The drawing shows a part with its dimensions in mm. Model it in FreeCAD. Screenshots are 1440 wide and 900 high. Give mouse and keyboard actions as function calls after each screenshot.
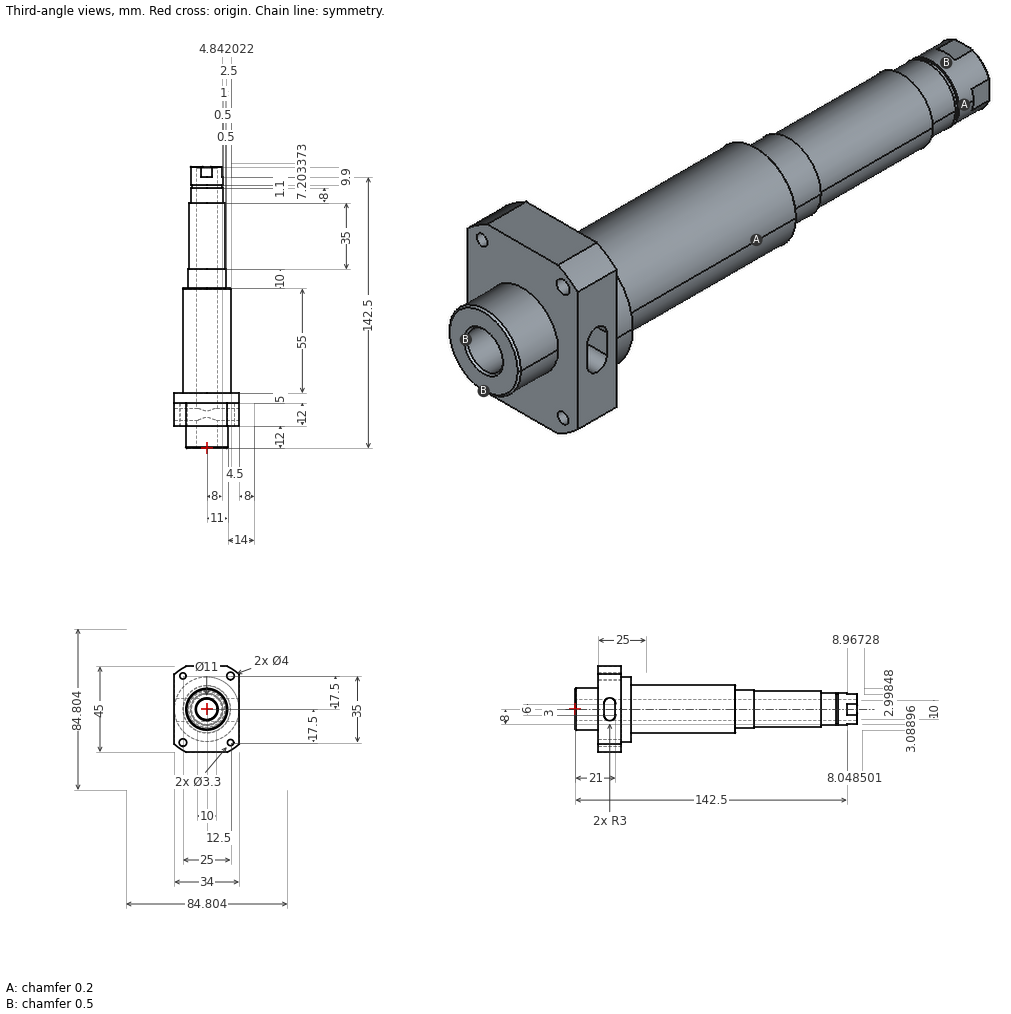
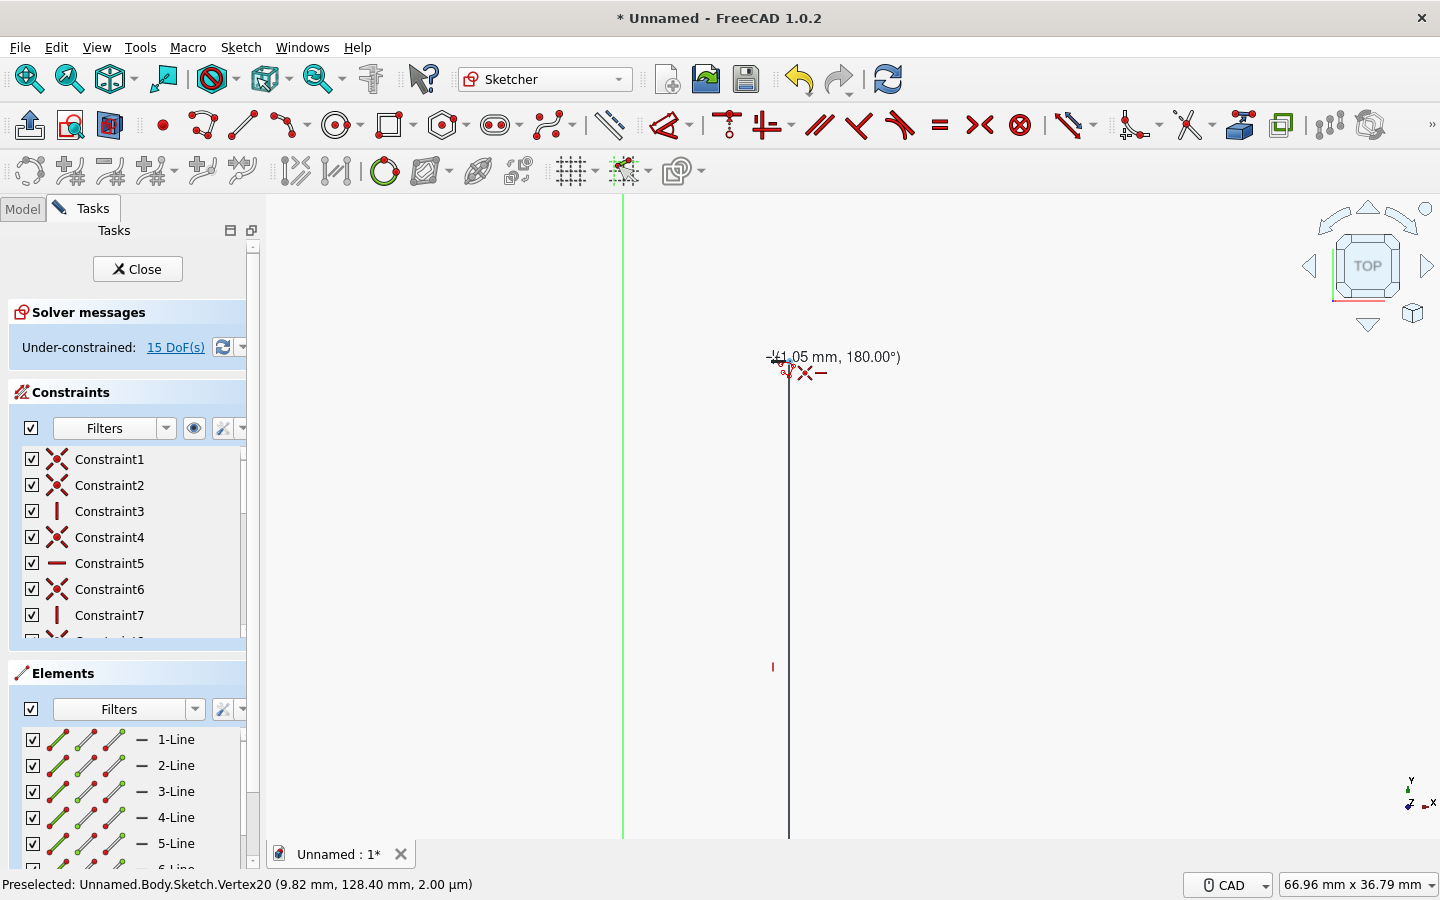
click(772, 356)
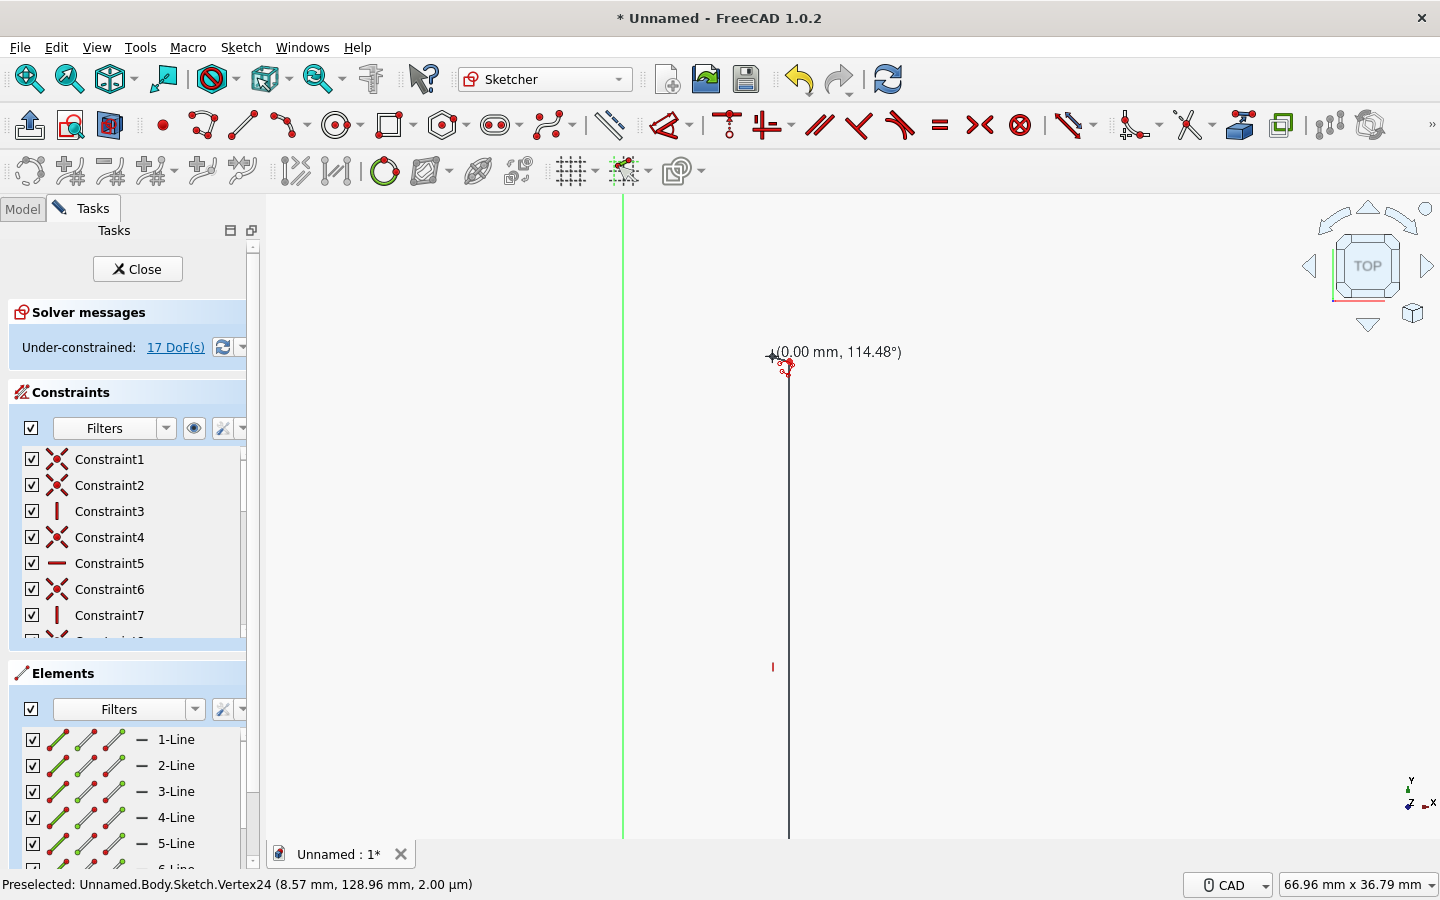
scroll(773, 357, down, 9)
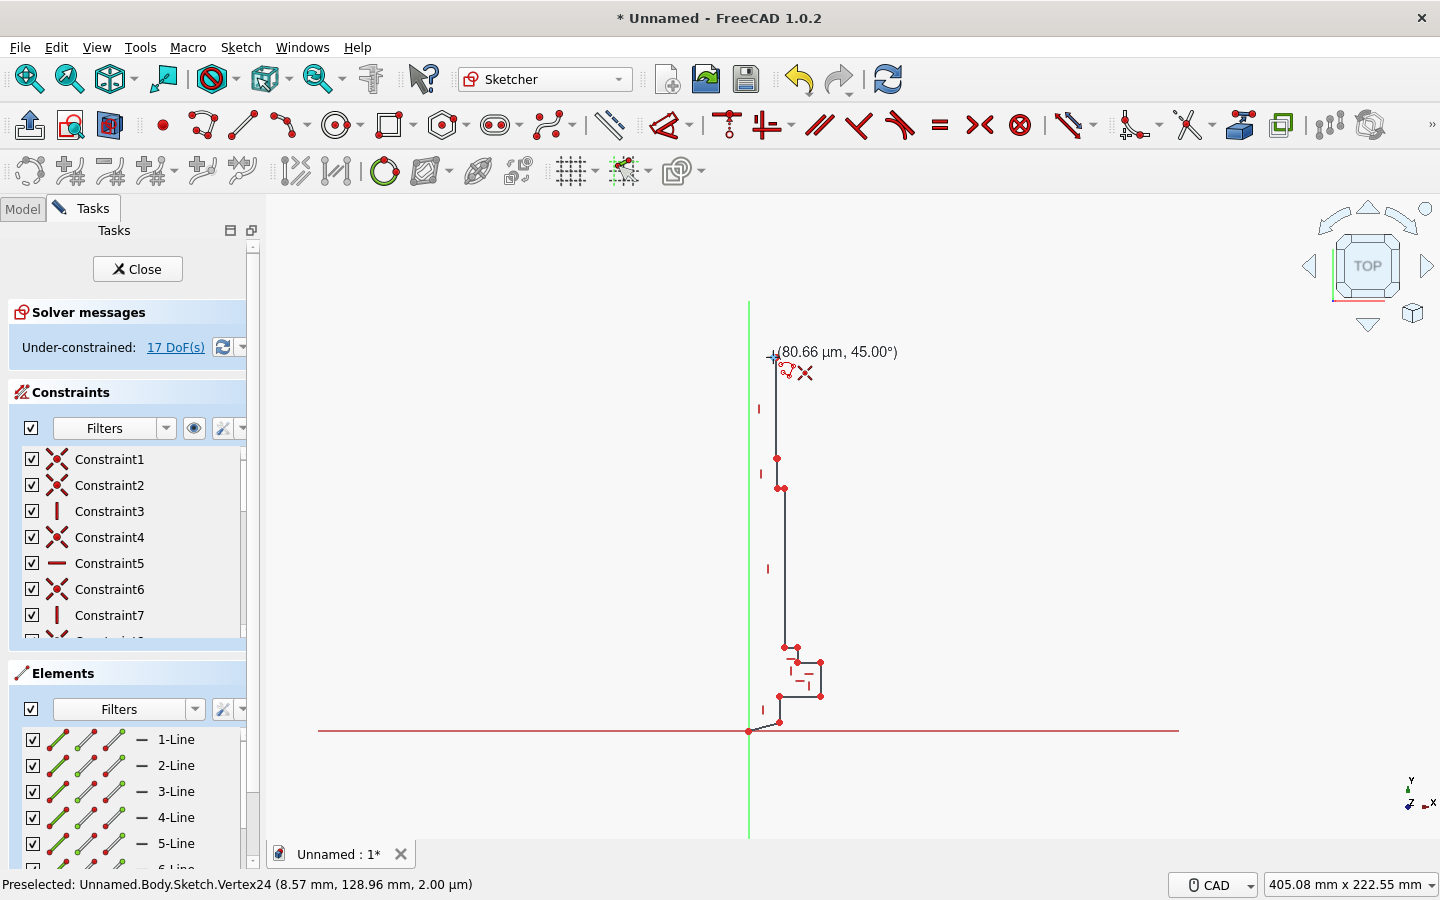
click(773, 334)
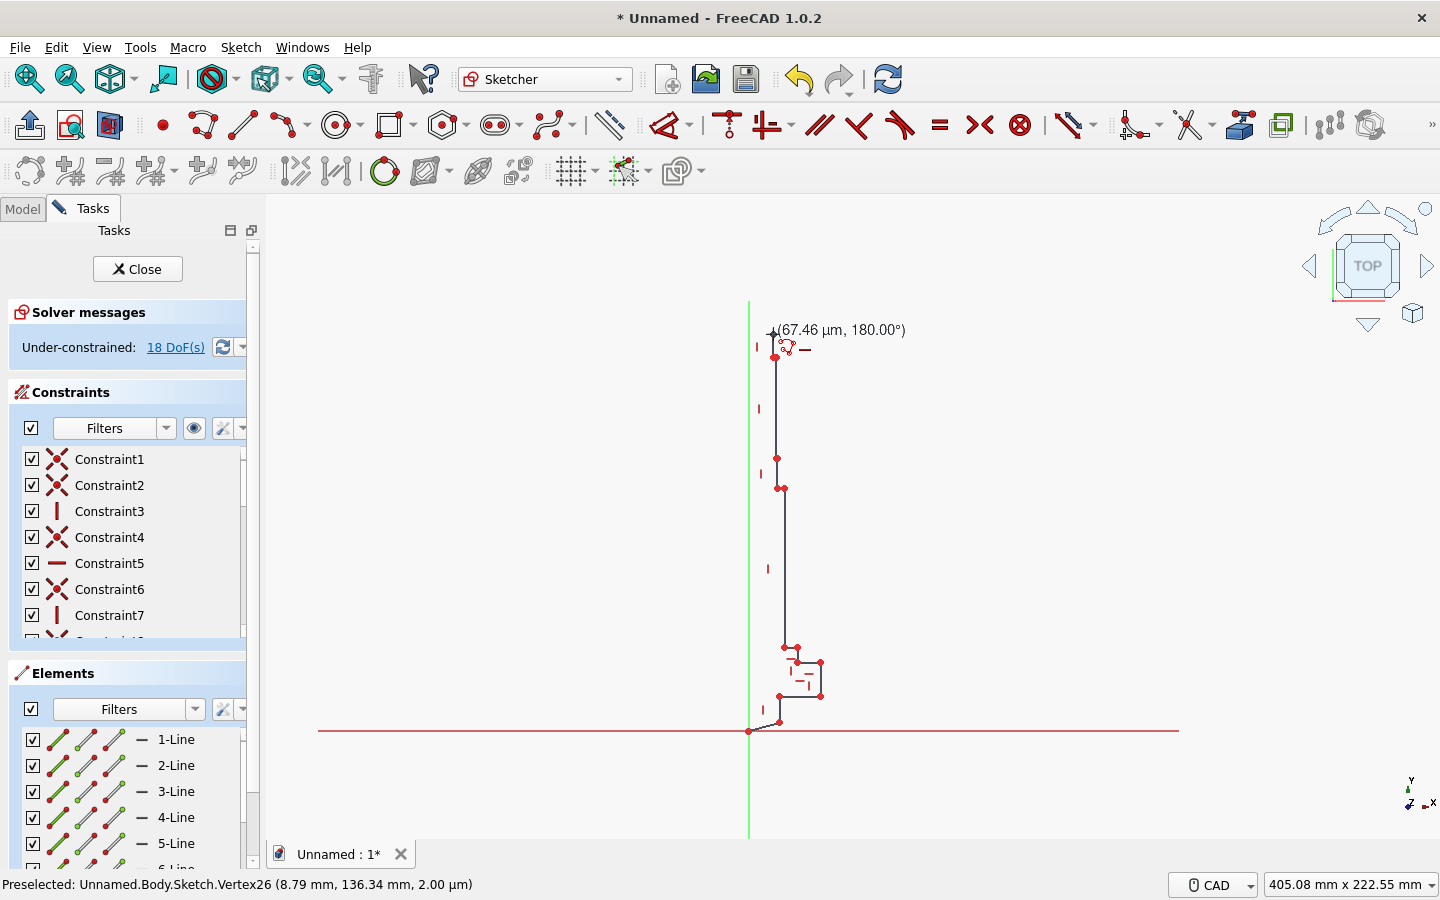
scroll(772, 334, up, 12)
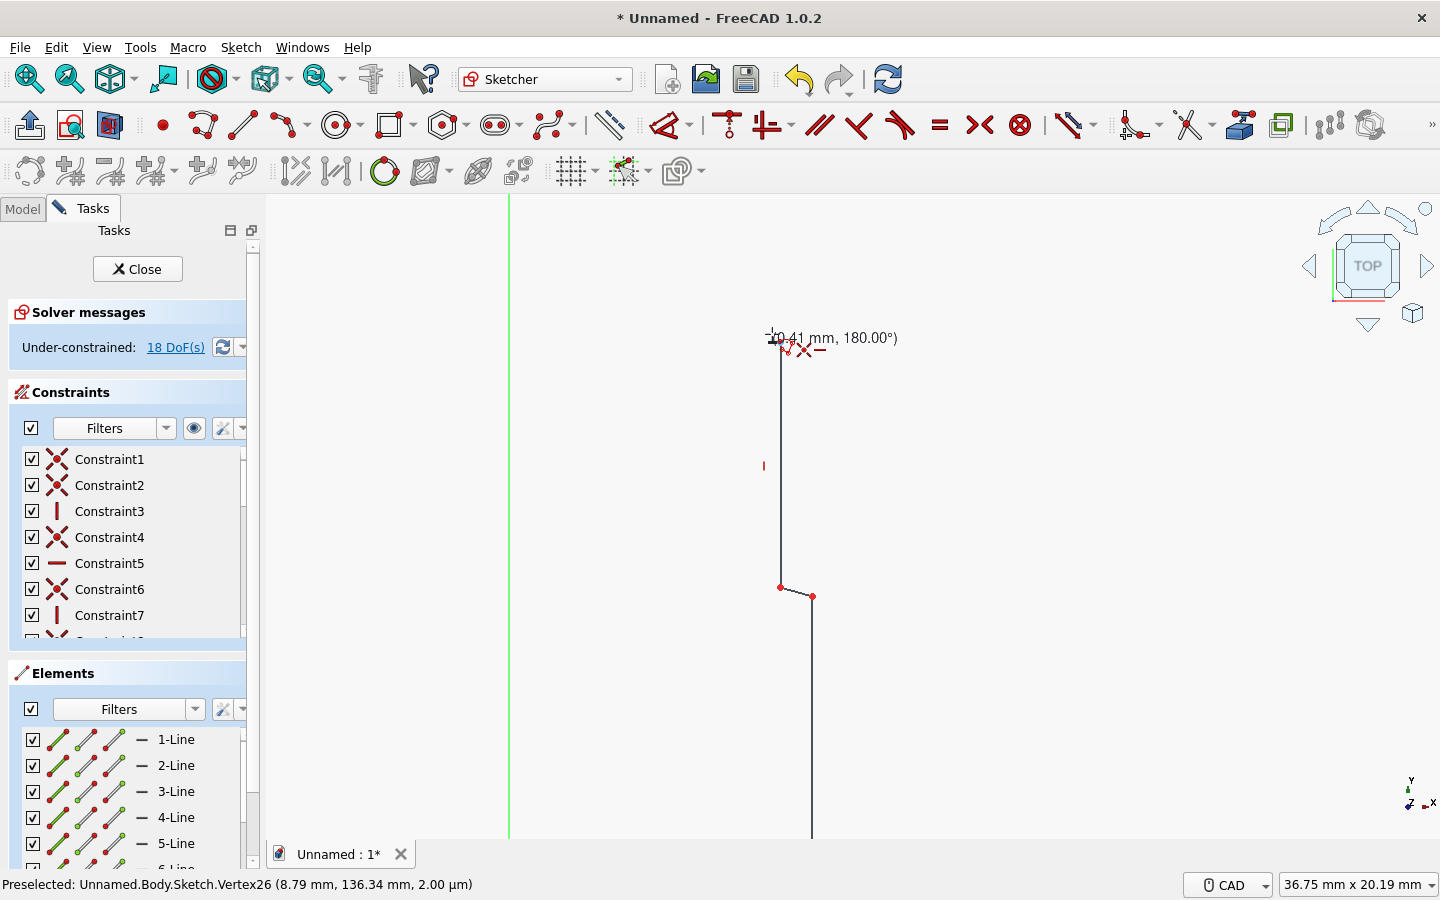
click(765, 332)
click(765, 298)
click(781, 298)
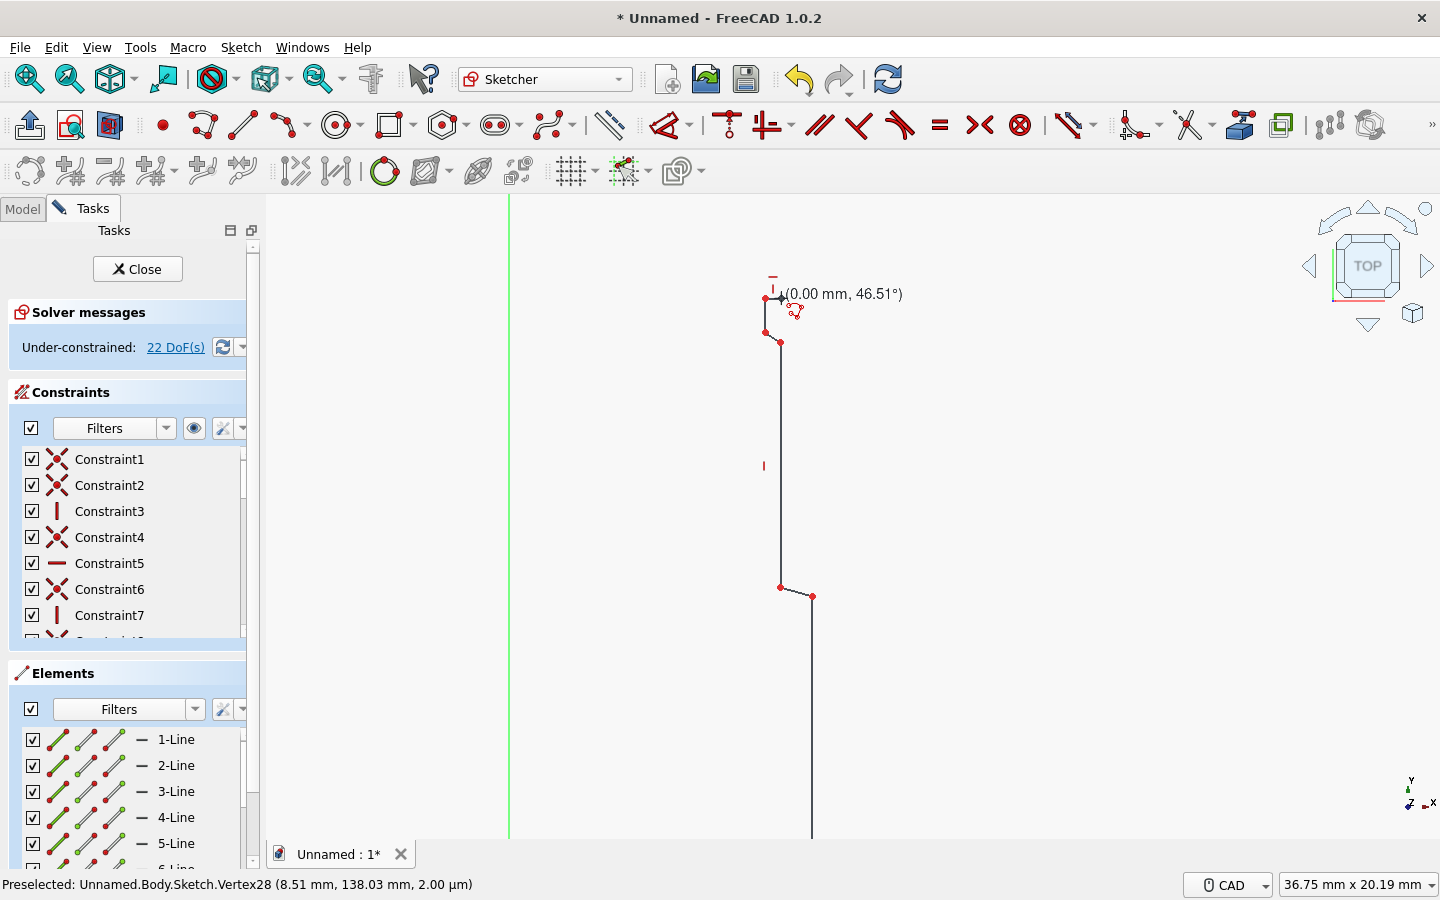
scroll(772, 334, down, 12)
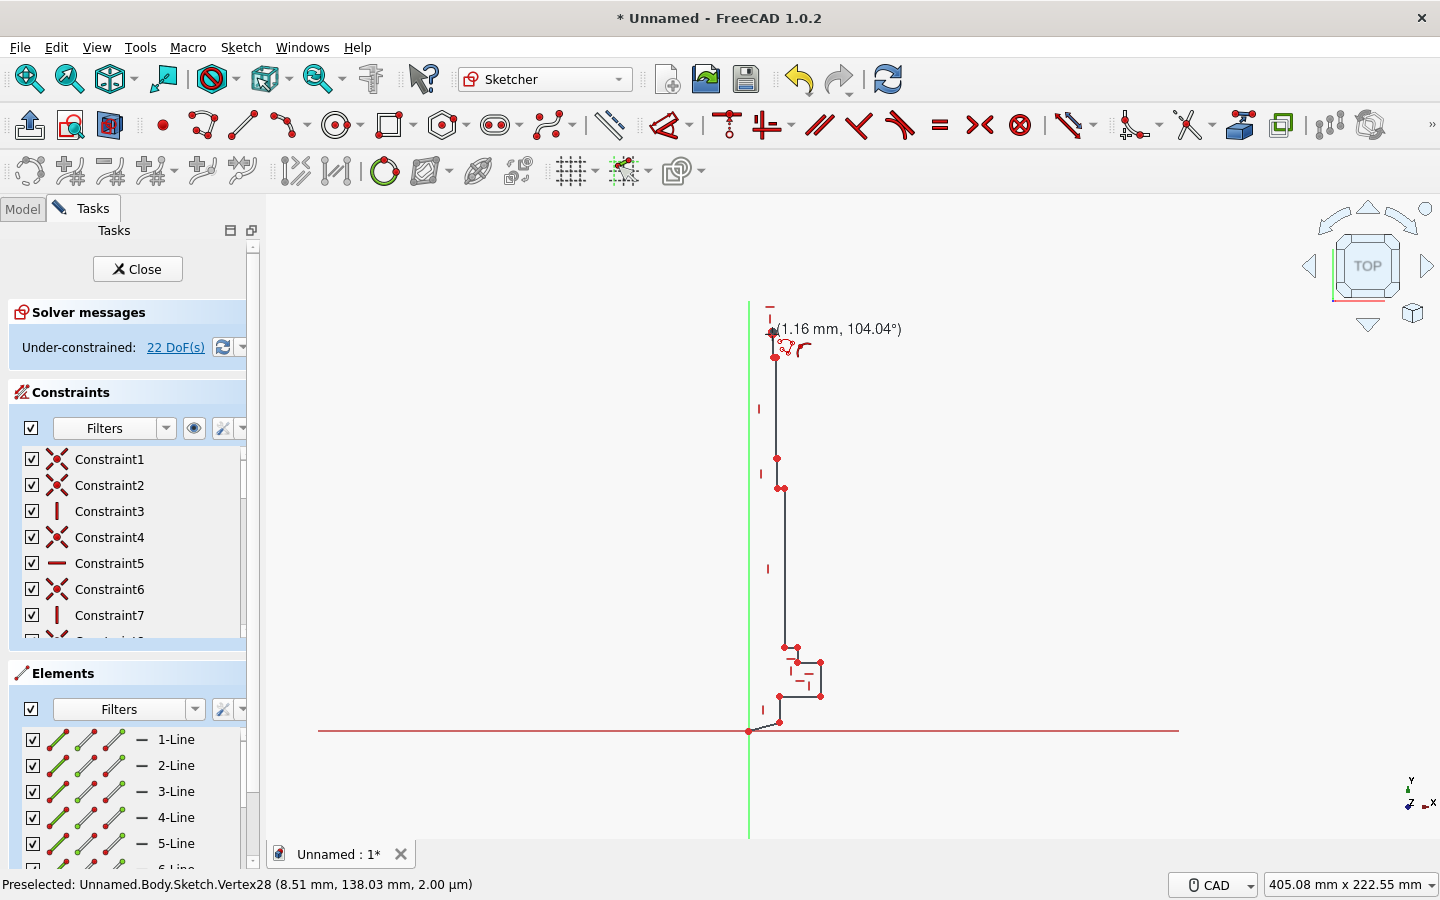
click(773, 302)
click(758, 302)
click(749, 731)
key(Escape)
key(Escape)